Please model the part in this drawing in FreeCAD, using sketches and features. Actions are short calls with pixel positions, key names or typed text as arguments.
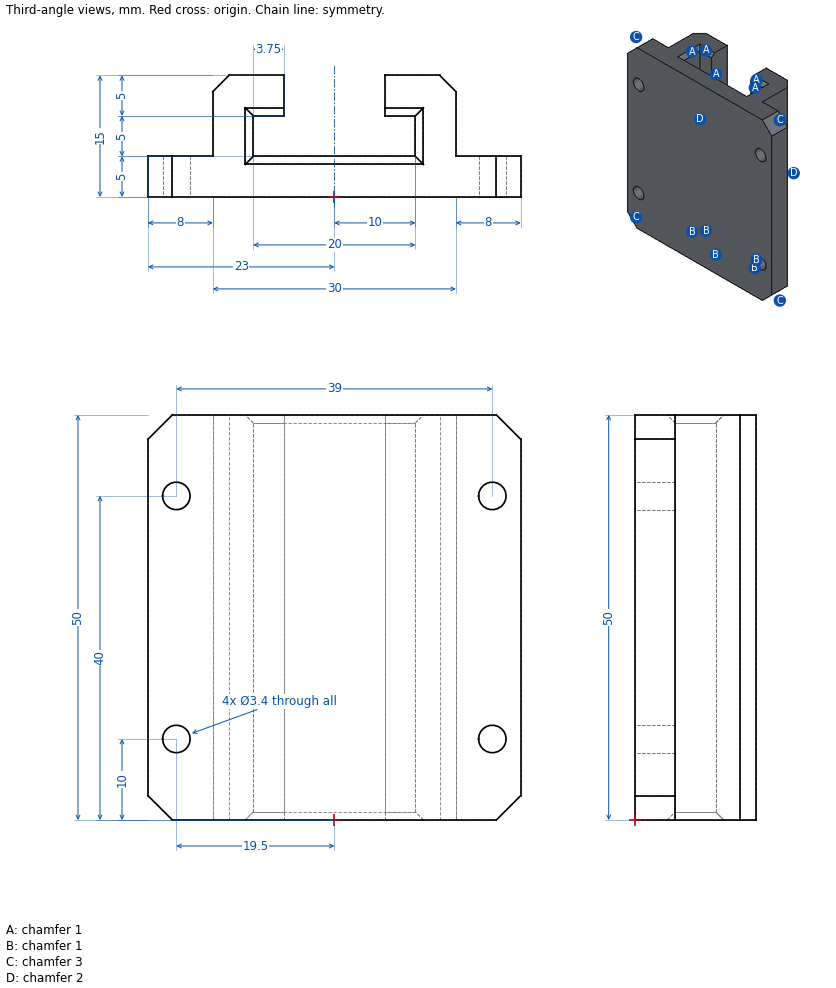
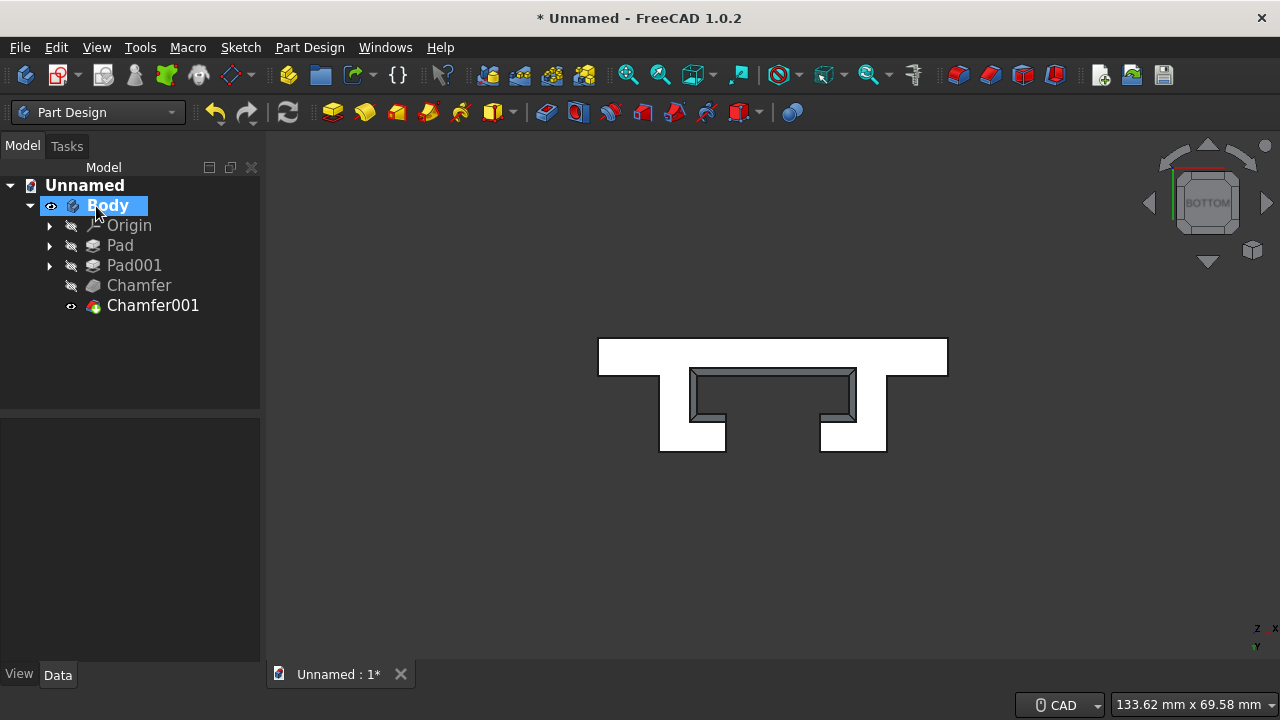
click(598, 356)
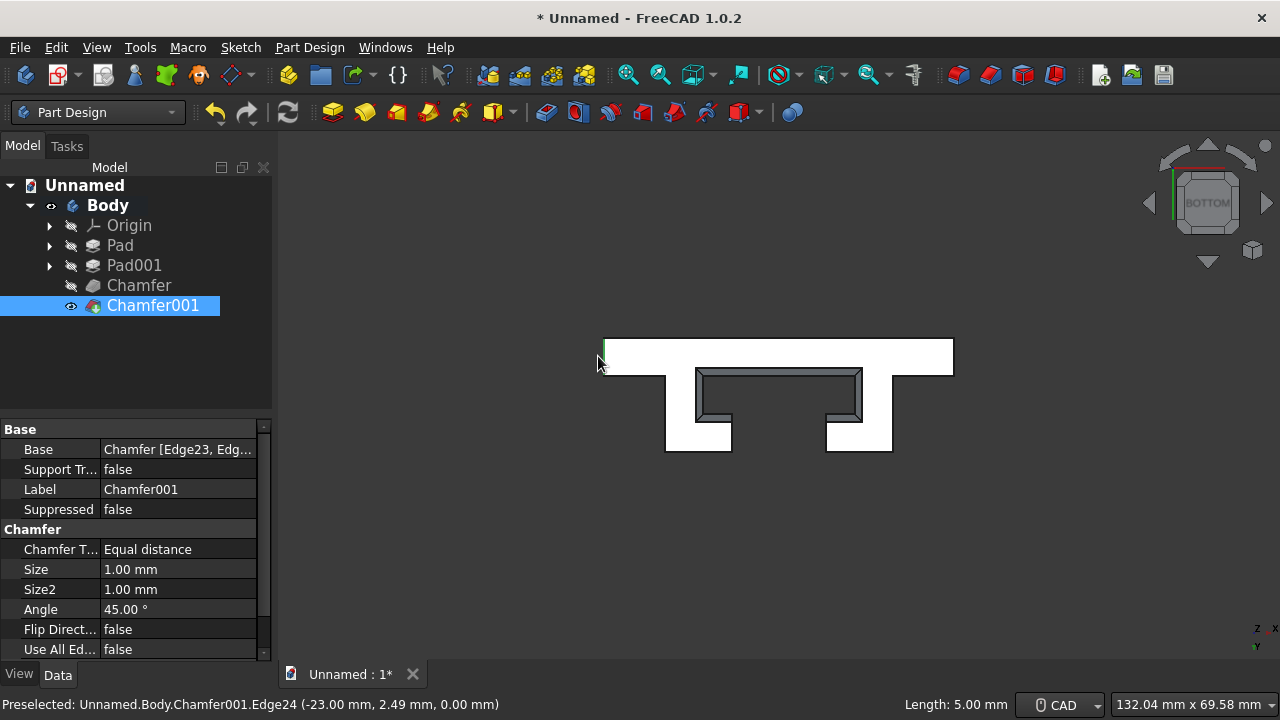
click(954, 356, ctrl)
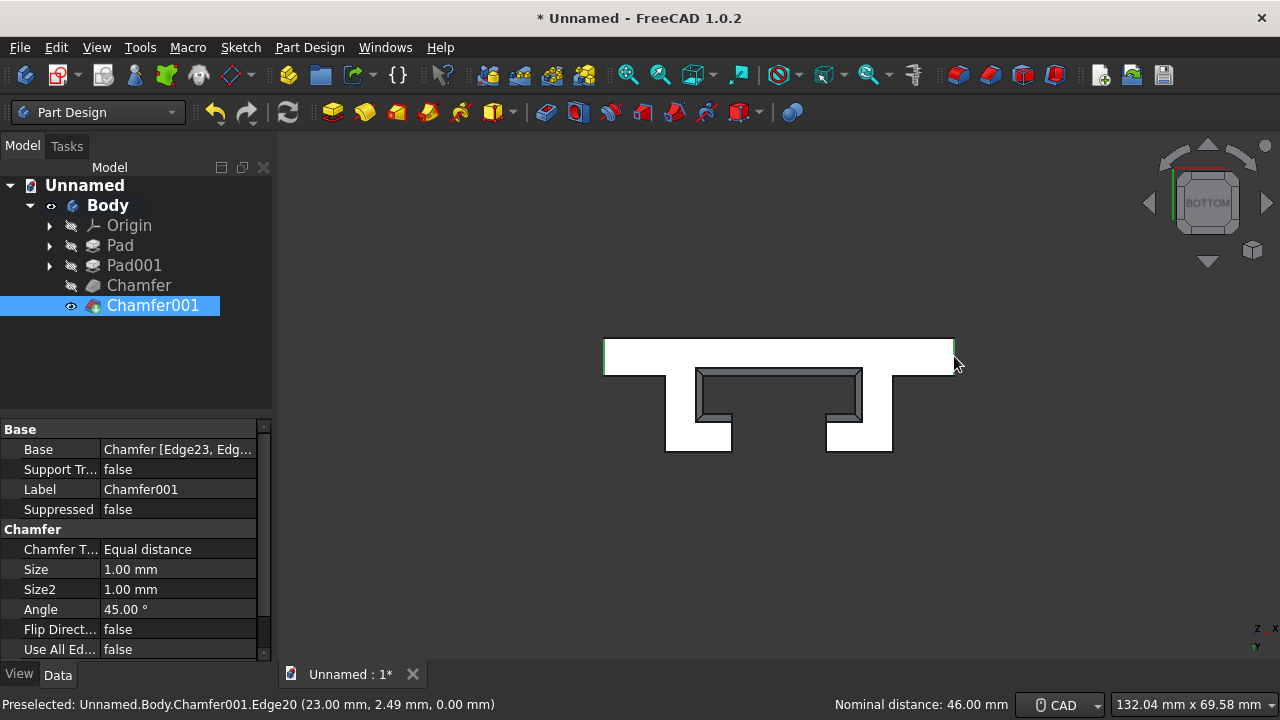
key(0)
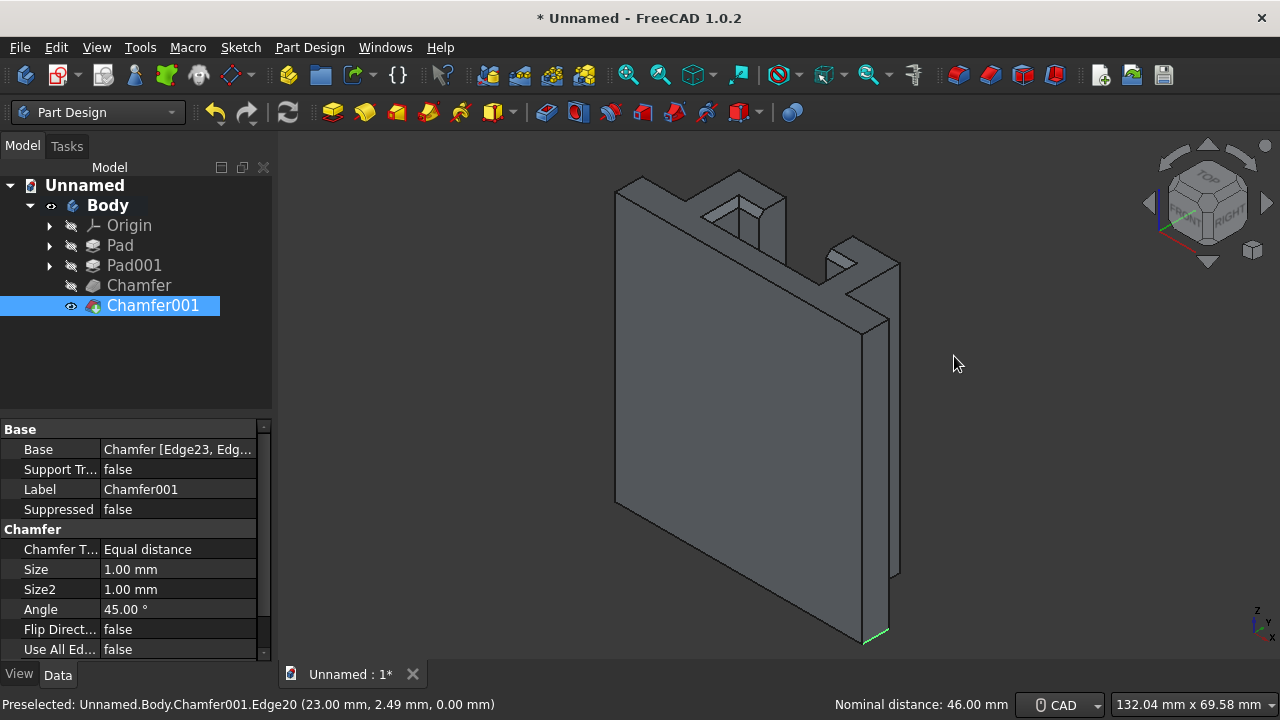
click(876, 326, ctrl)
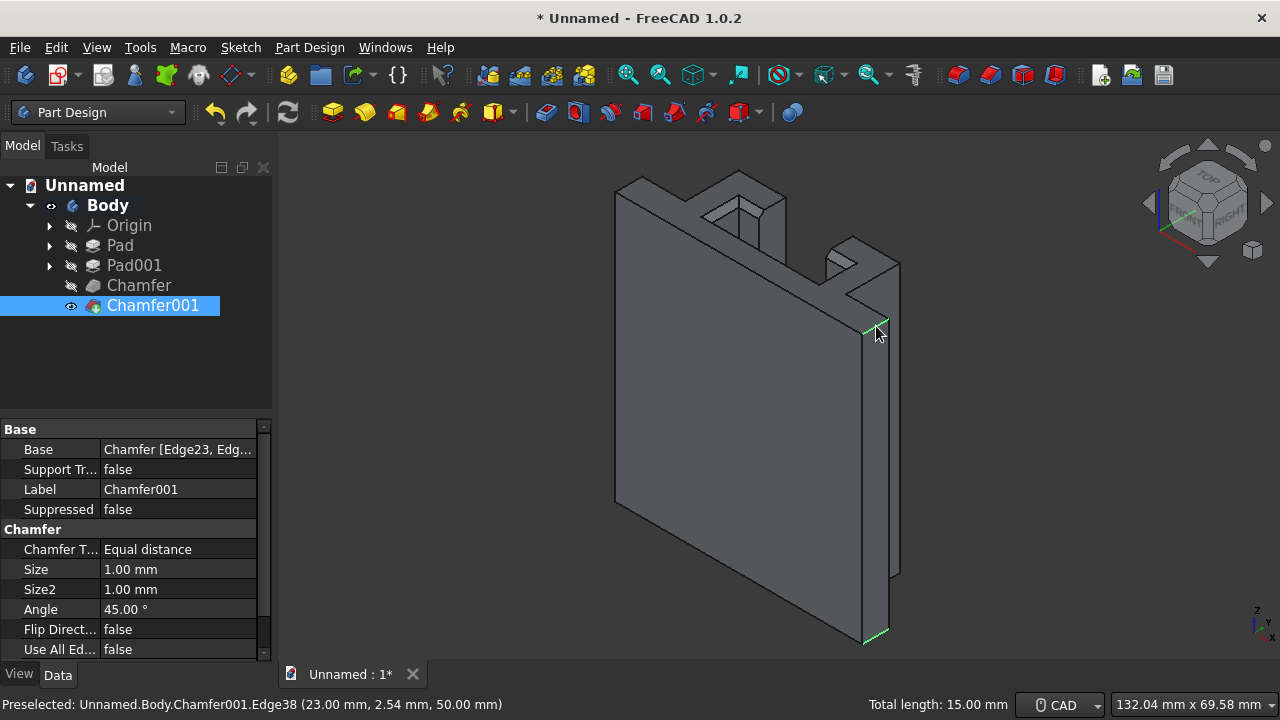
key(2)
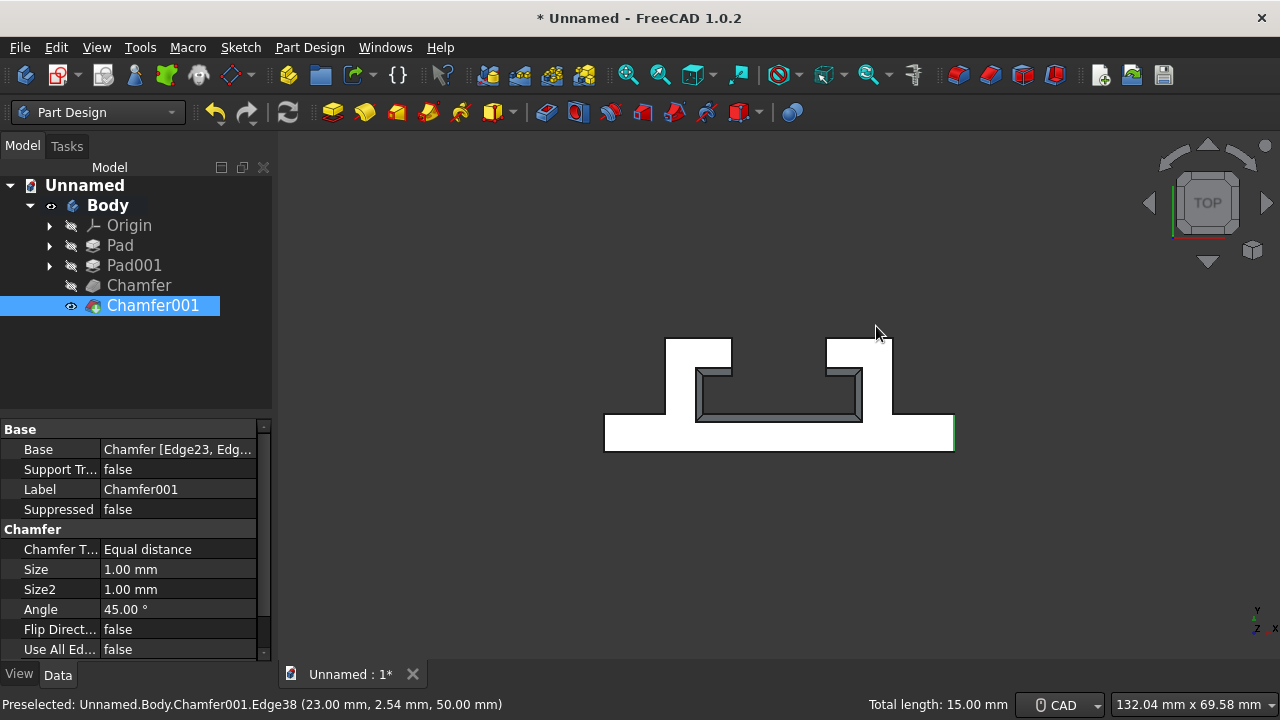
key(v)
key(f)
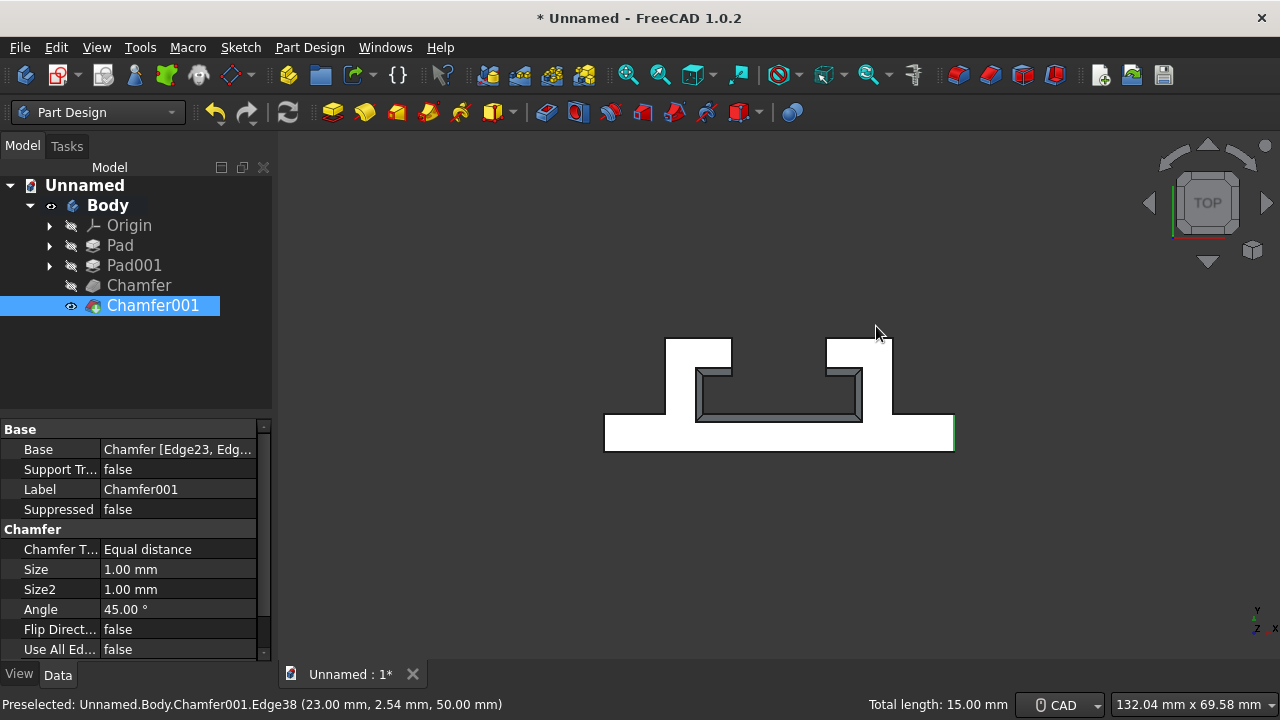
click(604, 432, ctrl)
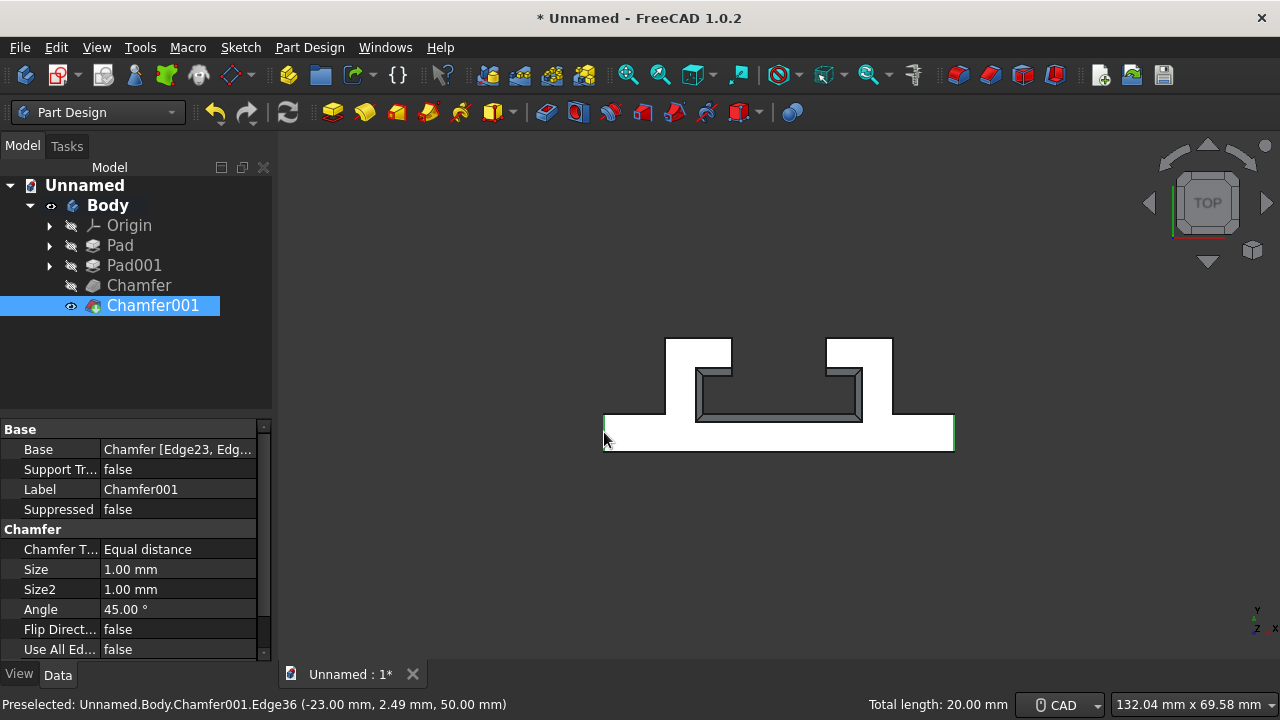
click(992, 76)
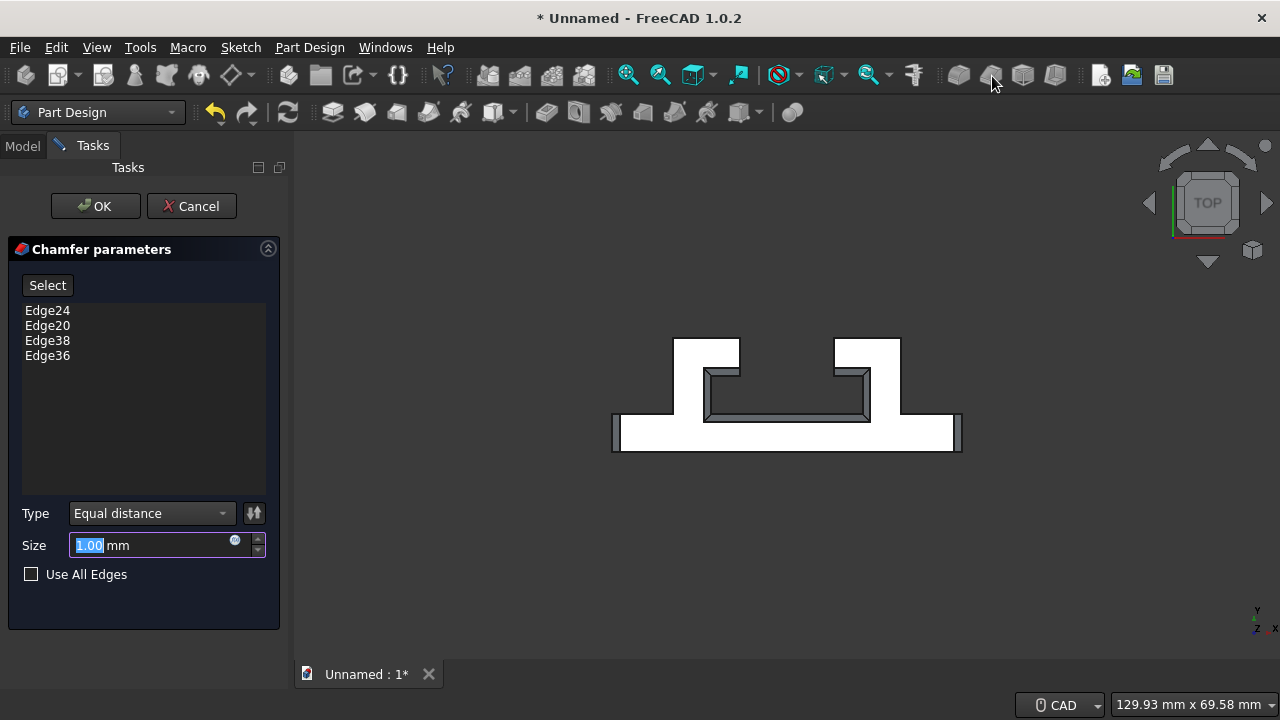
text(3)
key(Tab)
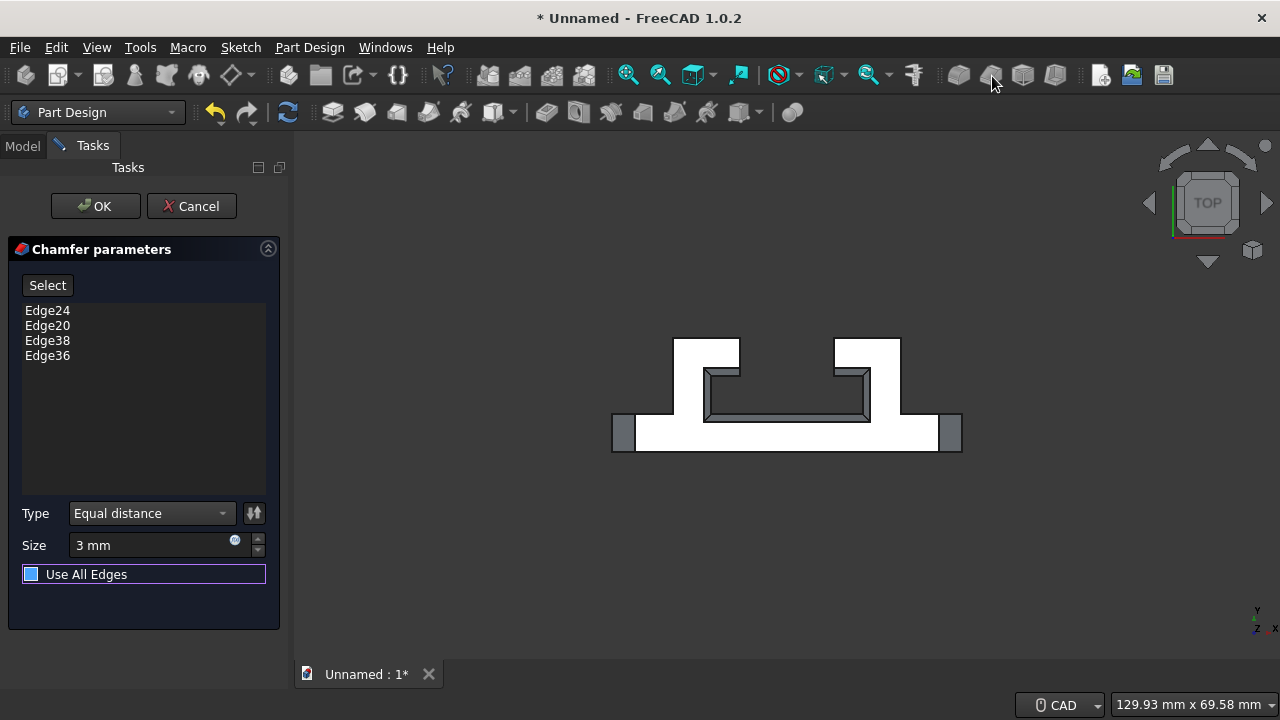
click(96, 206)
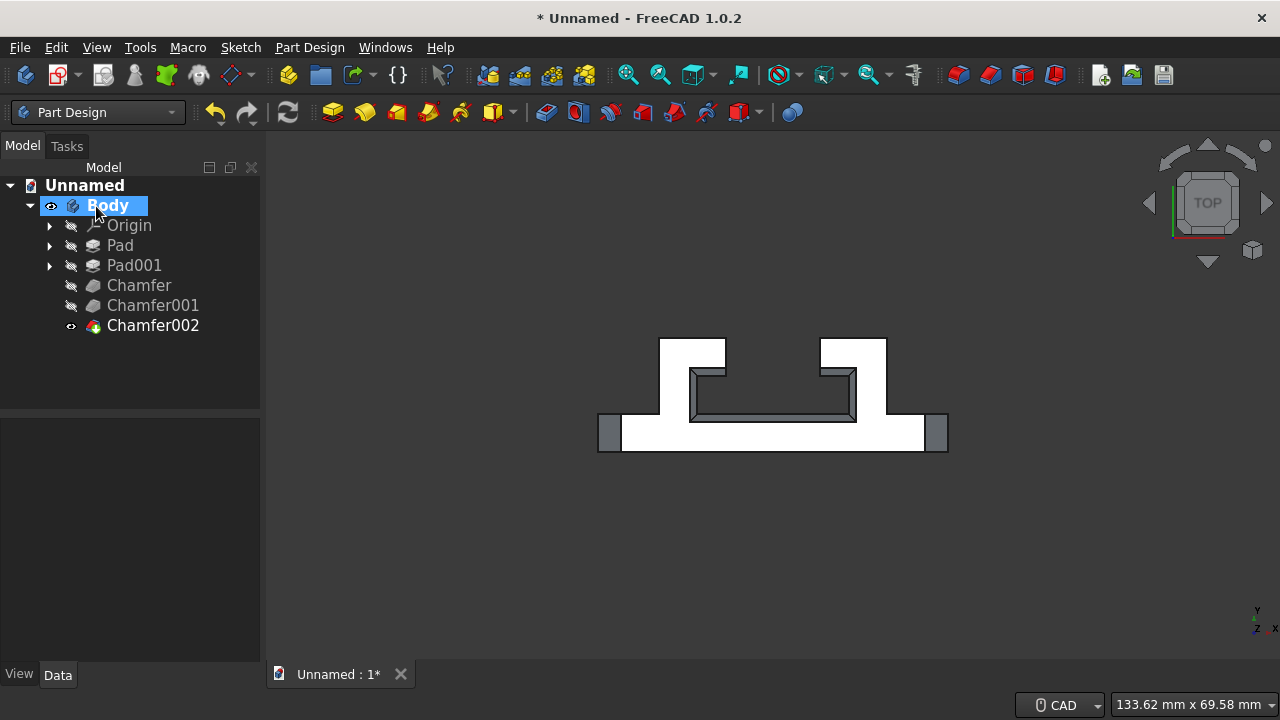
key(v)
key(f)